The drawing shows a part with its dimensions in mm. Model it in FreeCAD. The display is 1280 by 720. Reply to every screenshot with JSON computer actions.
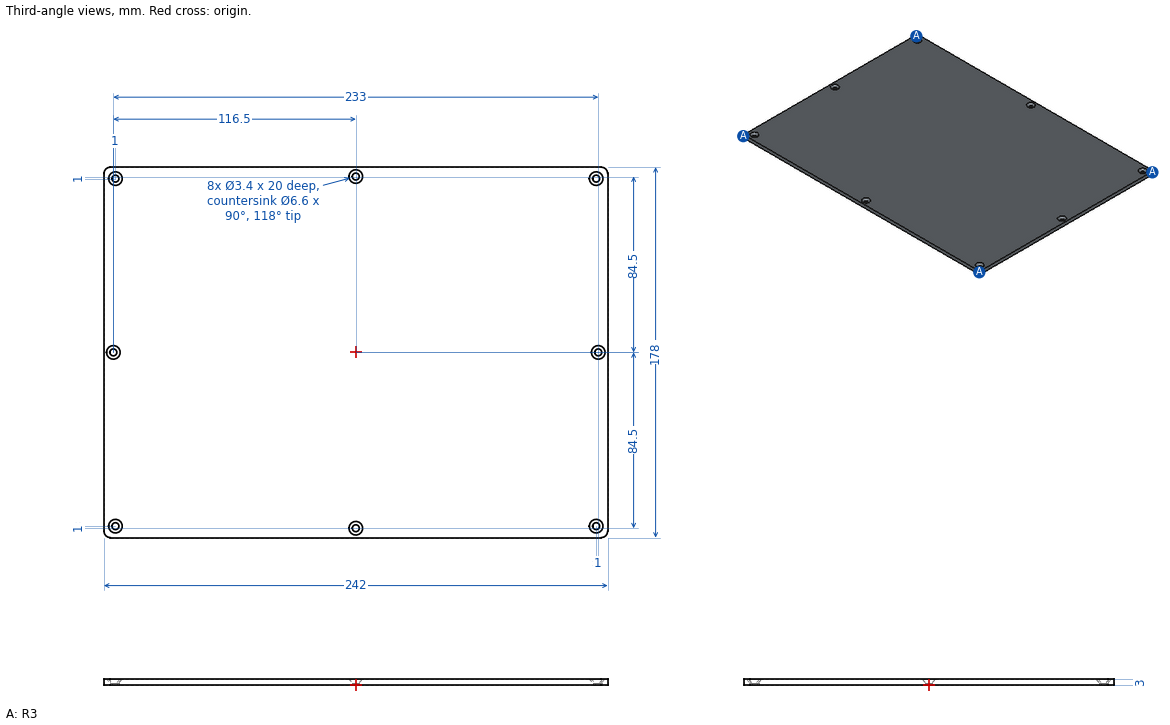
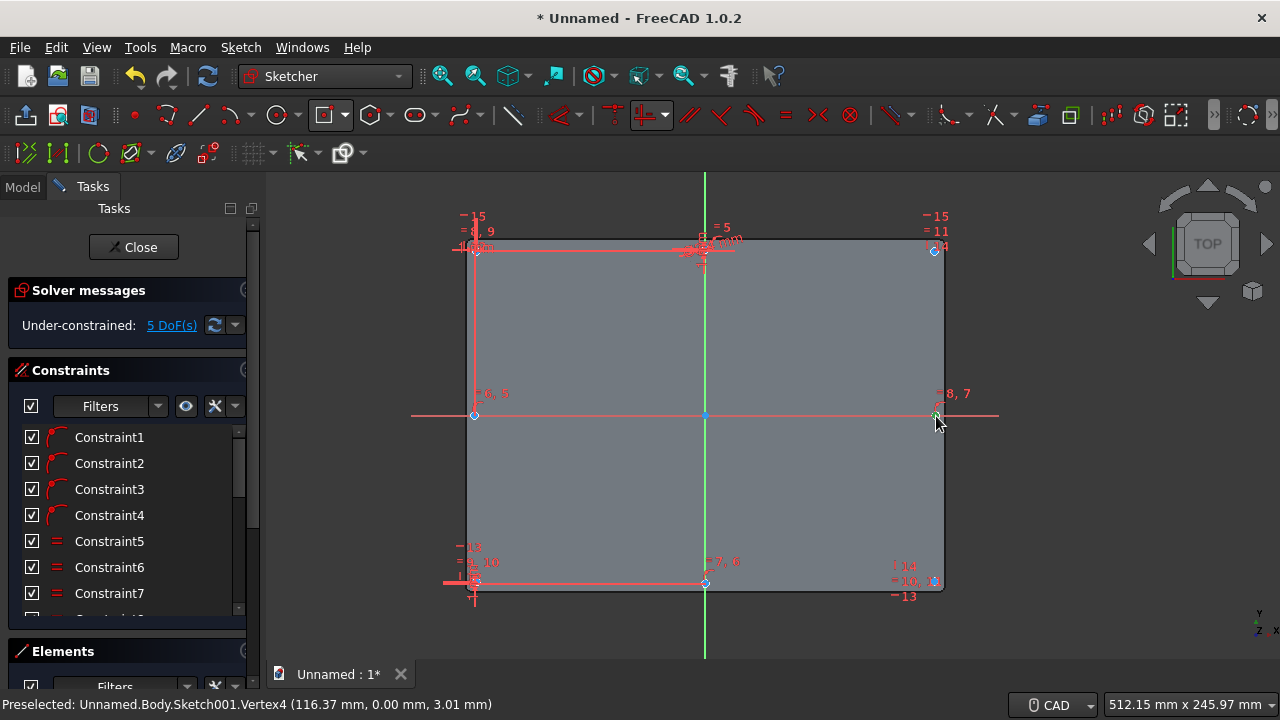
{"action": "scroll", "coordinate": [935, 582], "scroll_direction": "up", "scroll_amount": 15}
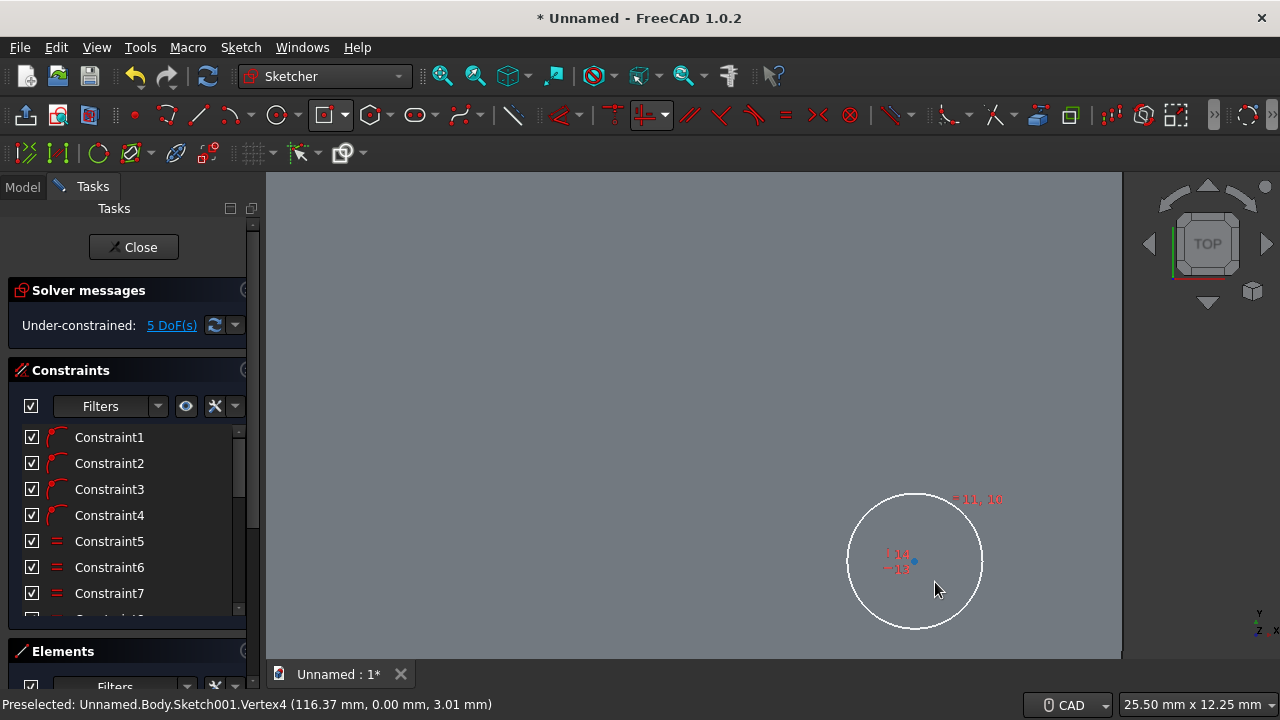
{"action": "left_click", "coordinate": [915, 561]}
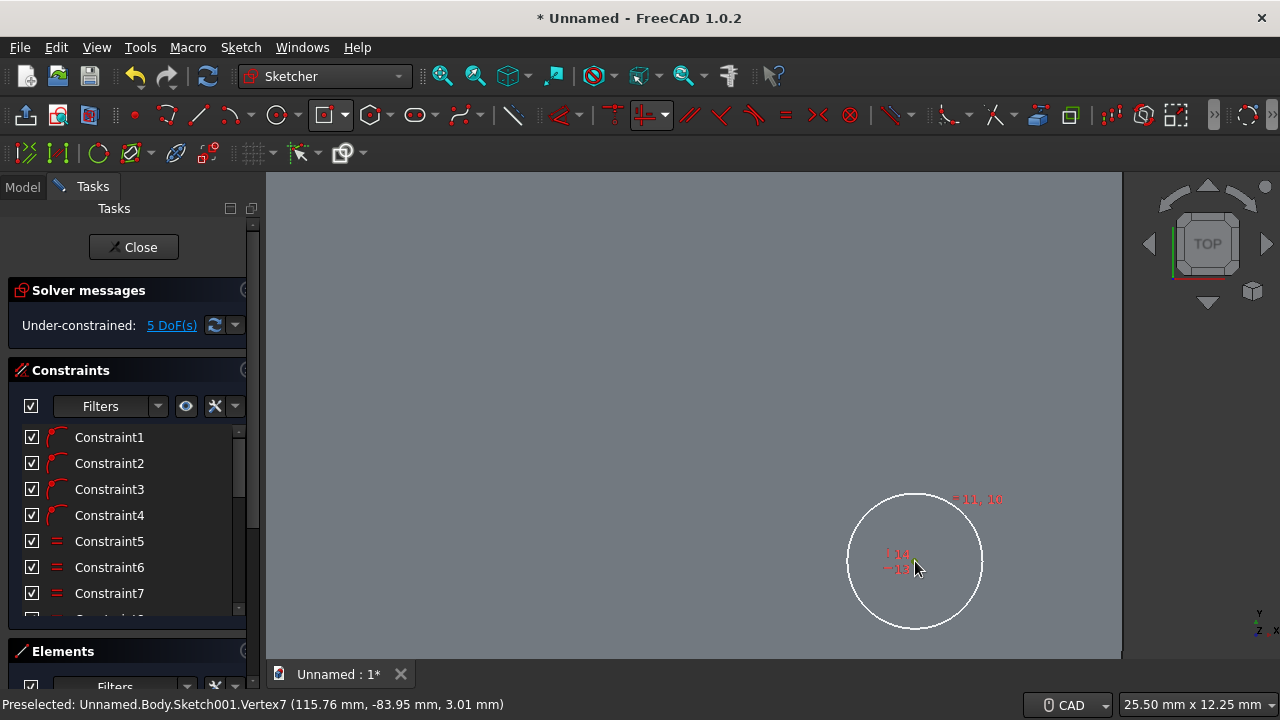
{"action": "key", "text": "l"}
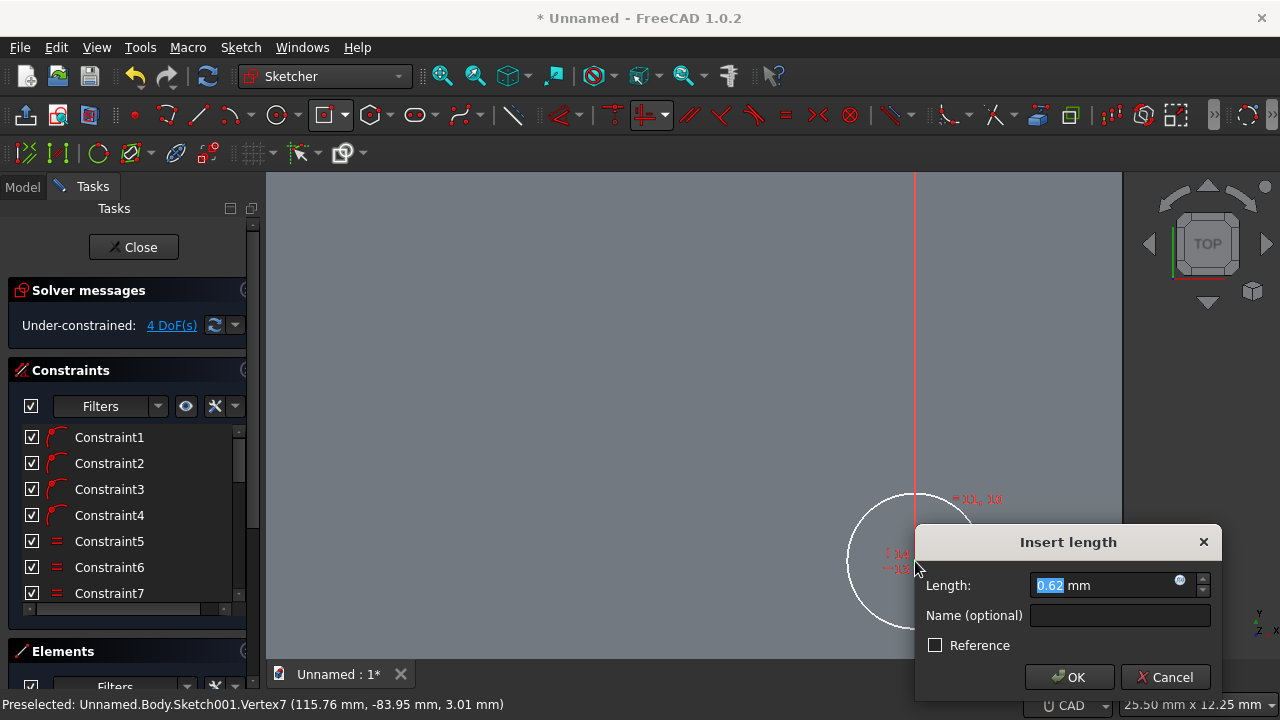
{"action": "type", "text": "1"}
{"action": "key", "text": "Return"}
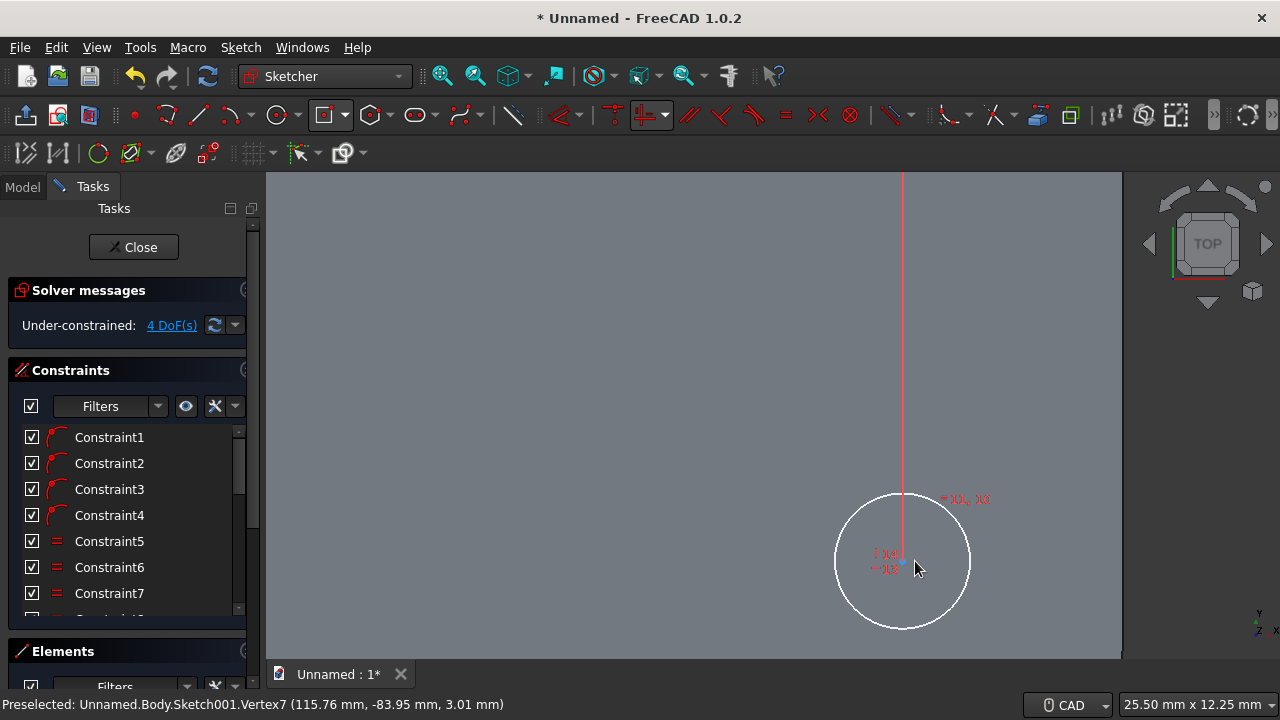
{"action": "scroll", "coordinate": [935, 583], "scroll_direction": "down", "scroll_amount": 15}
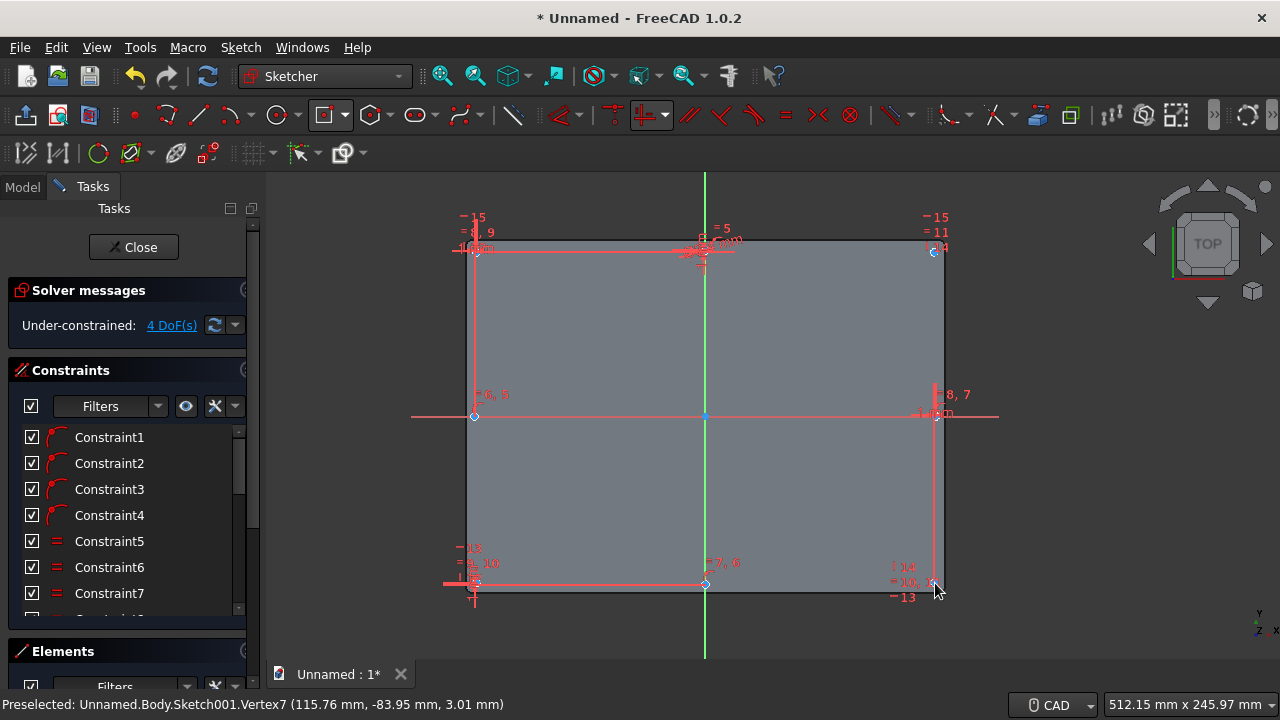
{"action": "left_click", "coordinate": [705, 250]}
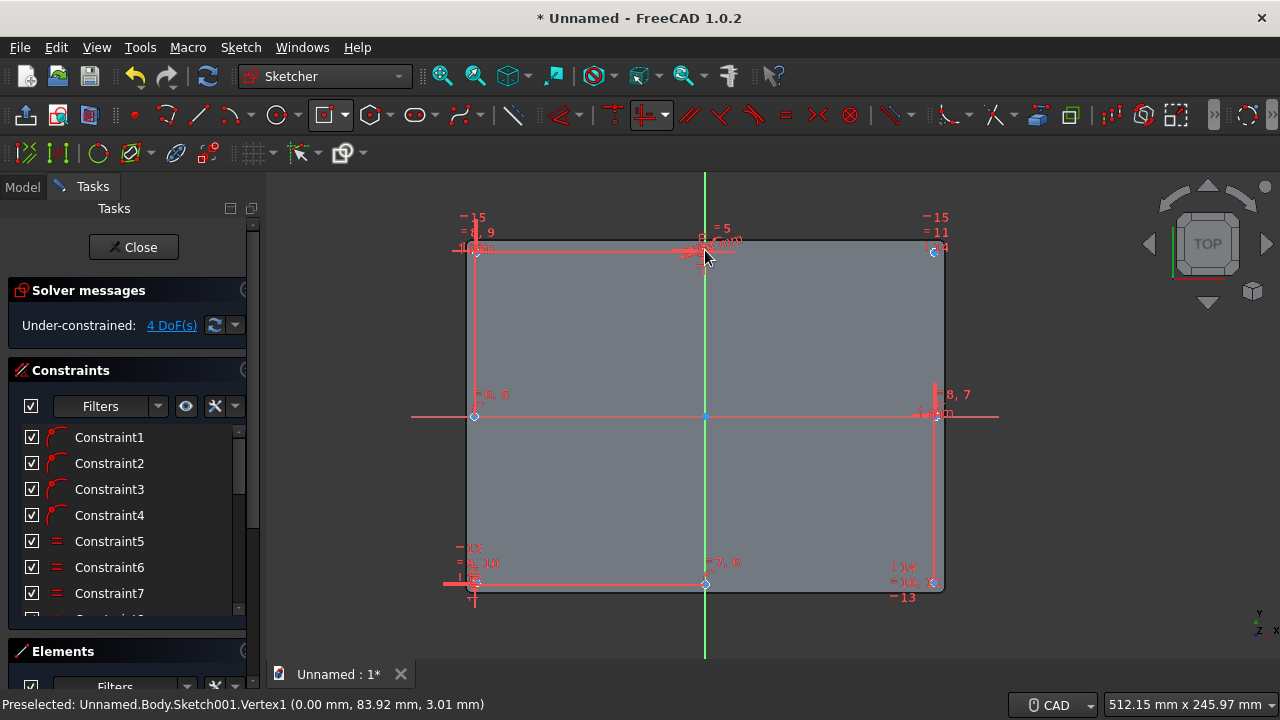
{"action": "key", "text": "i"}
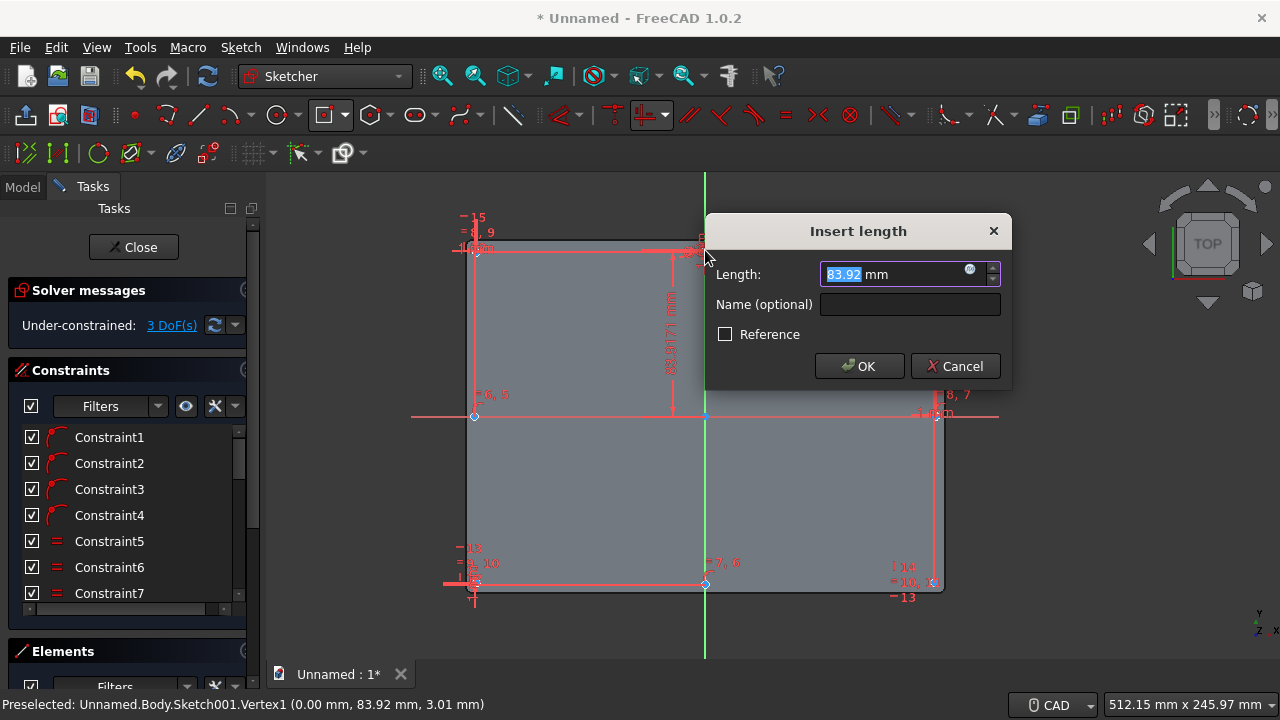
{"action": "type", "text": "84.5"}
{"action": "key", "text": "Return"}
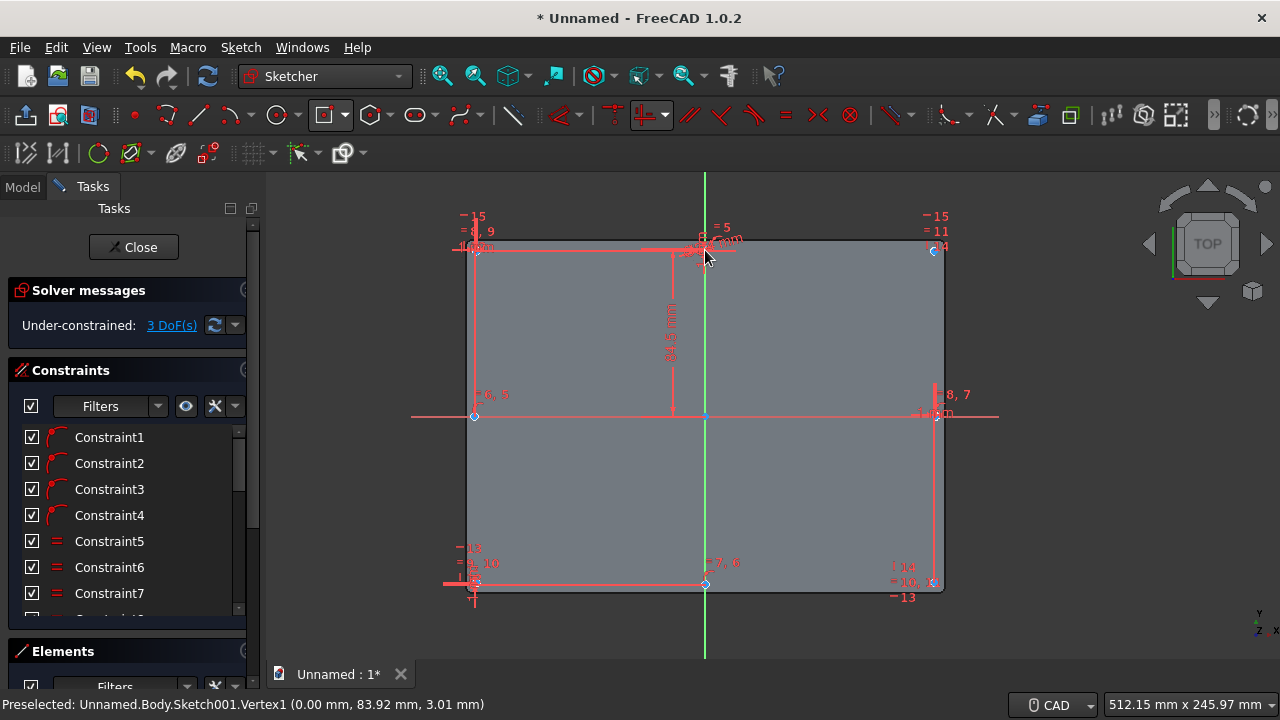
{"action": "left_click", "coordinate": [705, 585]}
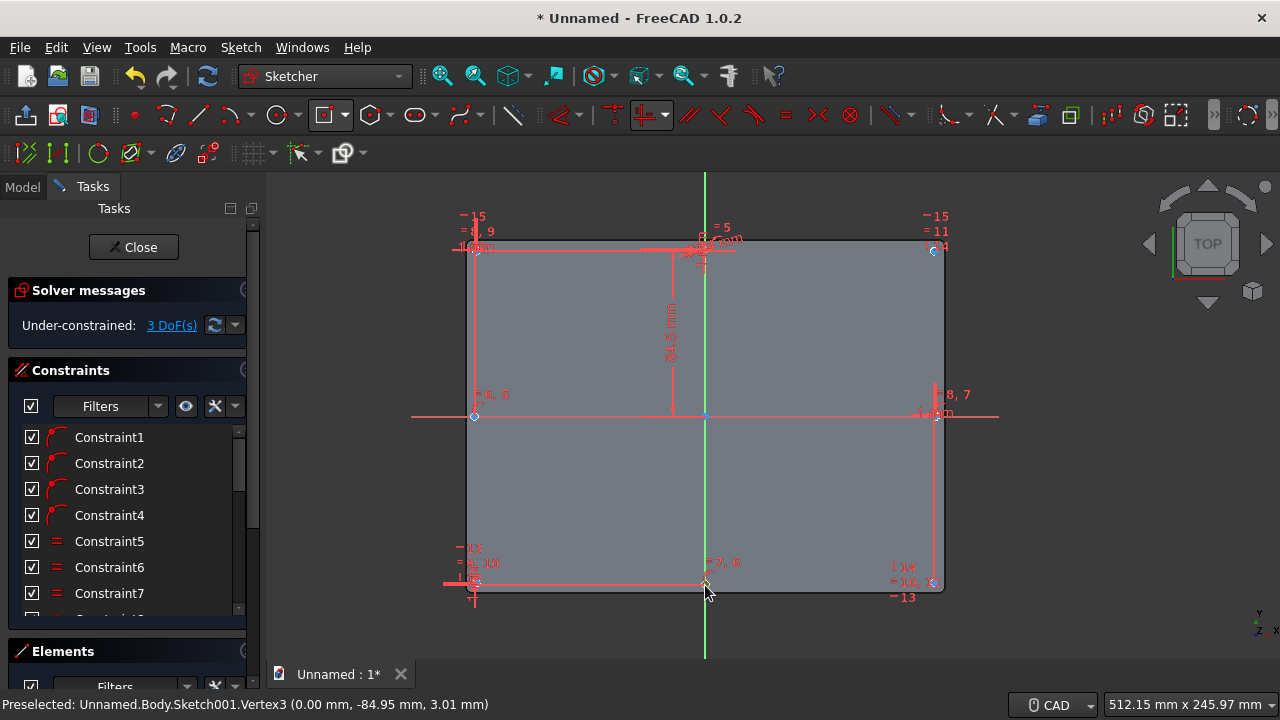
{"action": "left_click", "coordinate": [582, 116]}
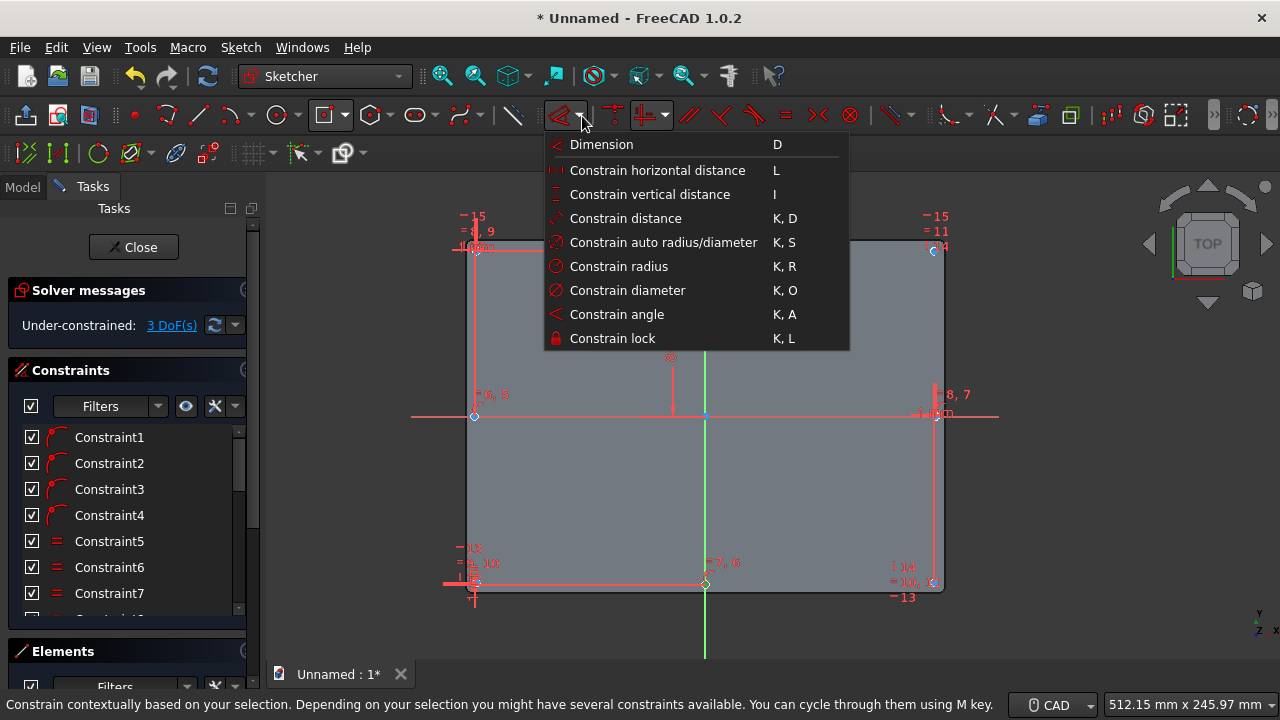
{"action": "left_click", "coordinate": [697, 194]}